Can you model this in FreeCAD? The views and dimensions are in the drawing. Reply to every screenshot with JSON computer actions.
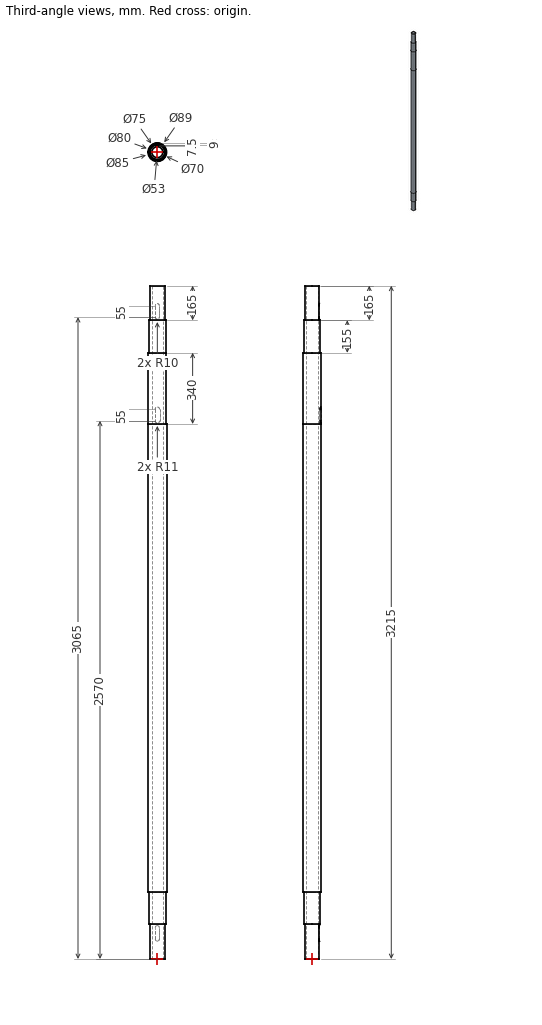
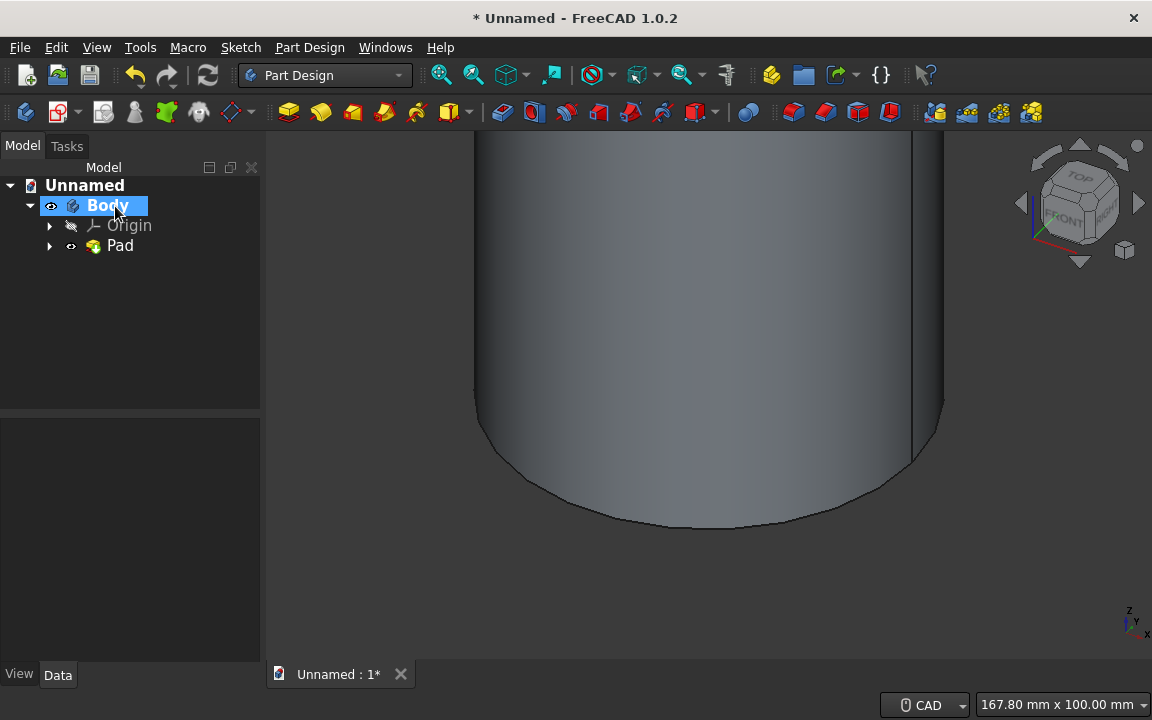
{"action": "left_click", "coordinate": [442, 76]}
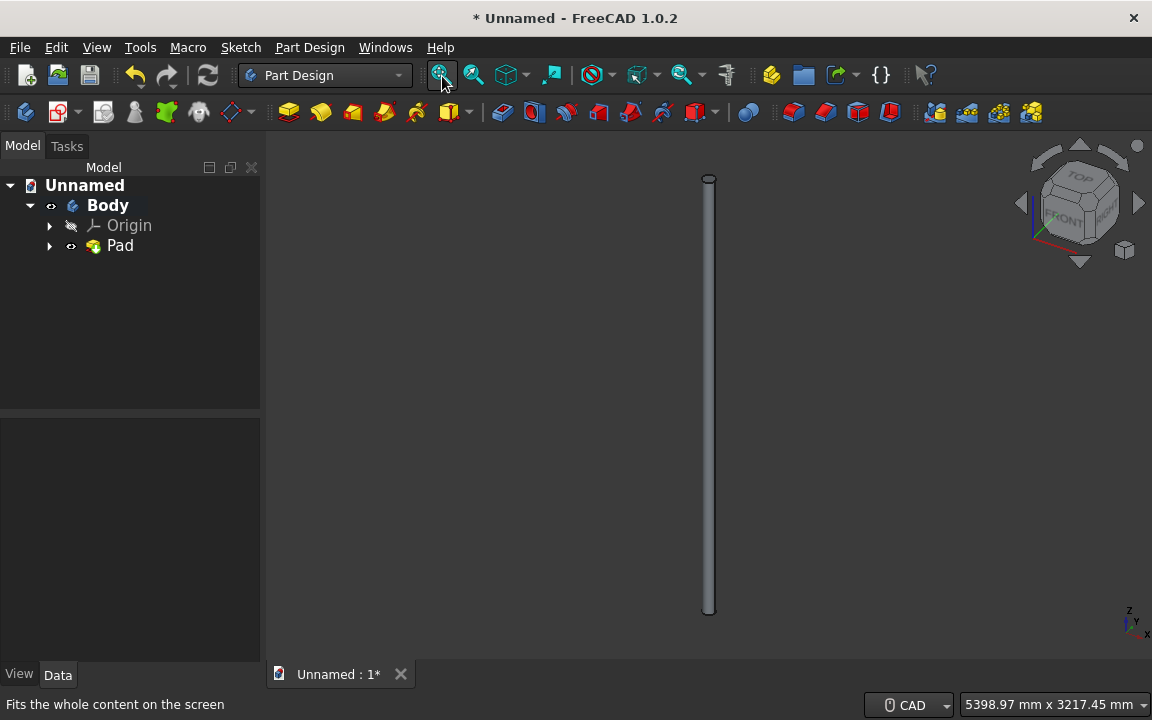
{"action": "left_click", "coordinate": [50, 226]}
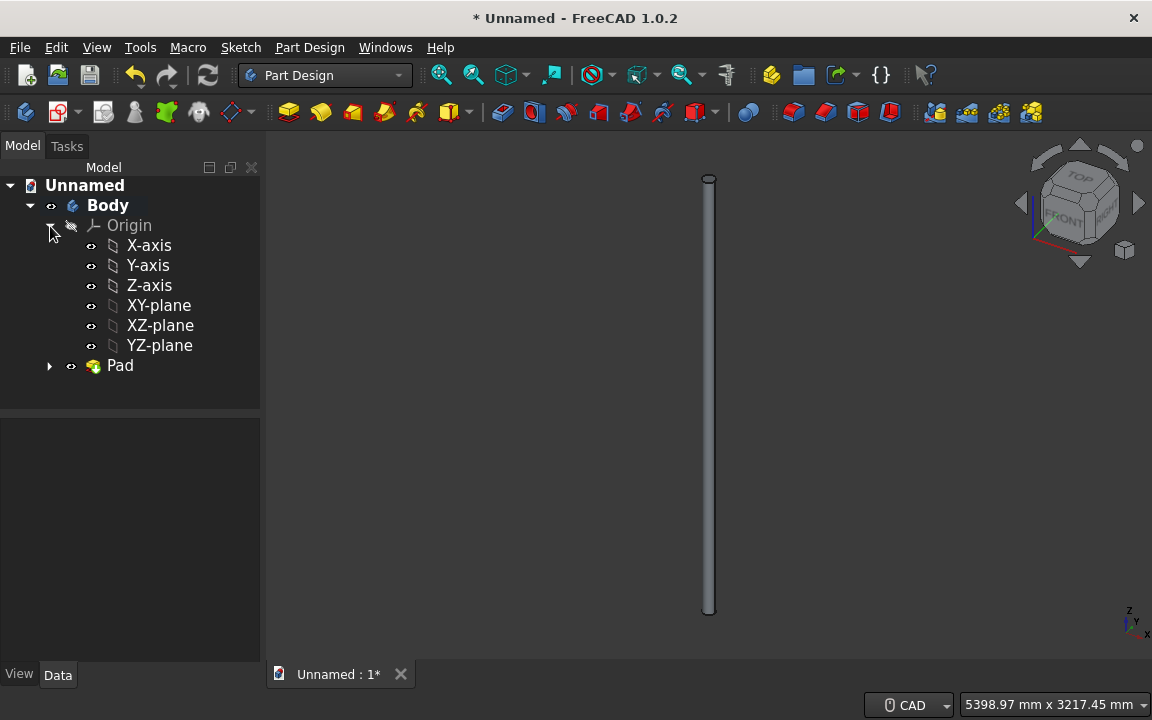
{"action": "left_click", "coordinate": [136, 306]}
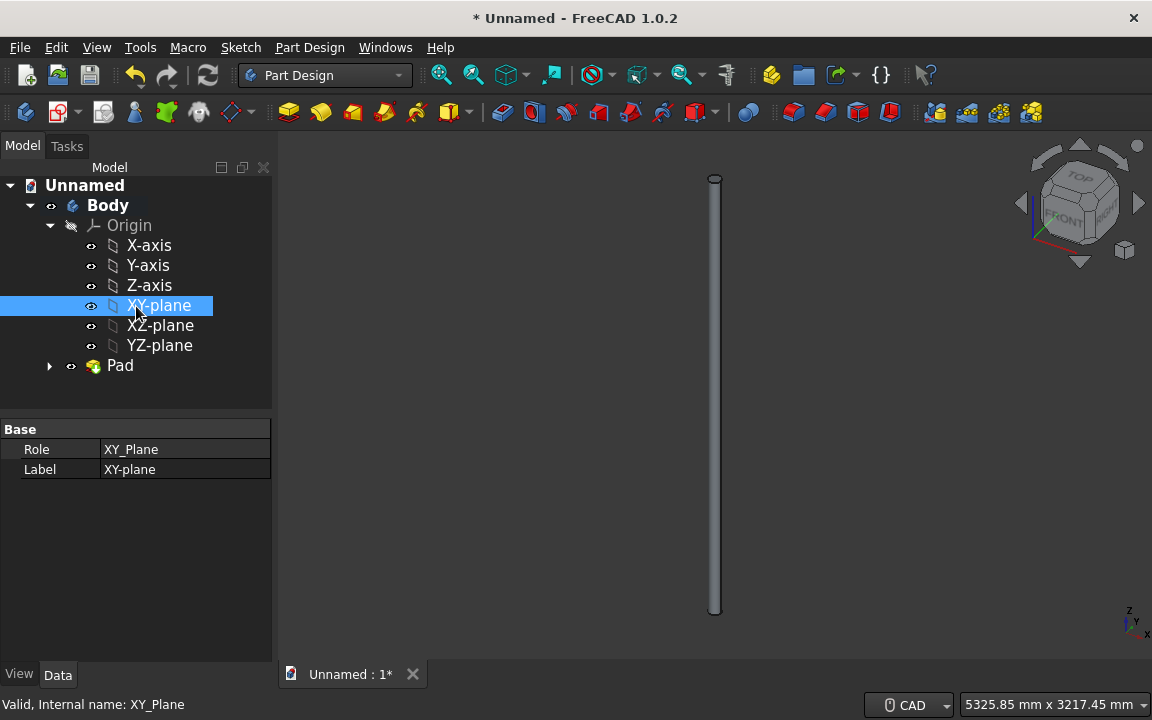
{"action": "left_click", "coordinate": [232, 112]}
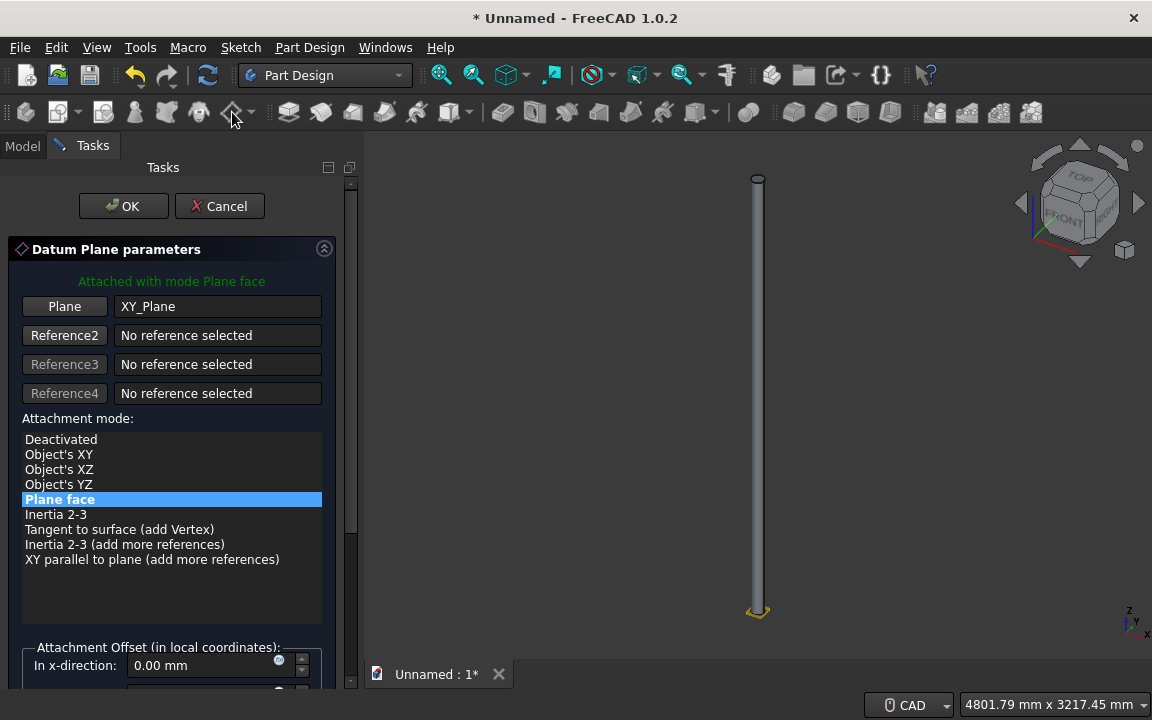
{"action": "scroll", "coordinate": [351, 432], "scroll_direction": "down", "scroll_amount": 2}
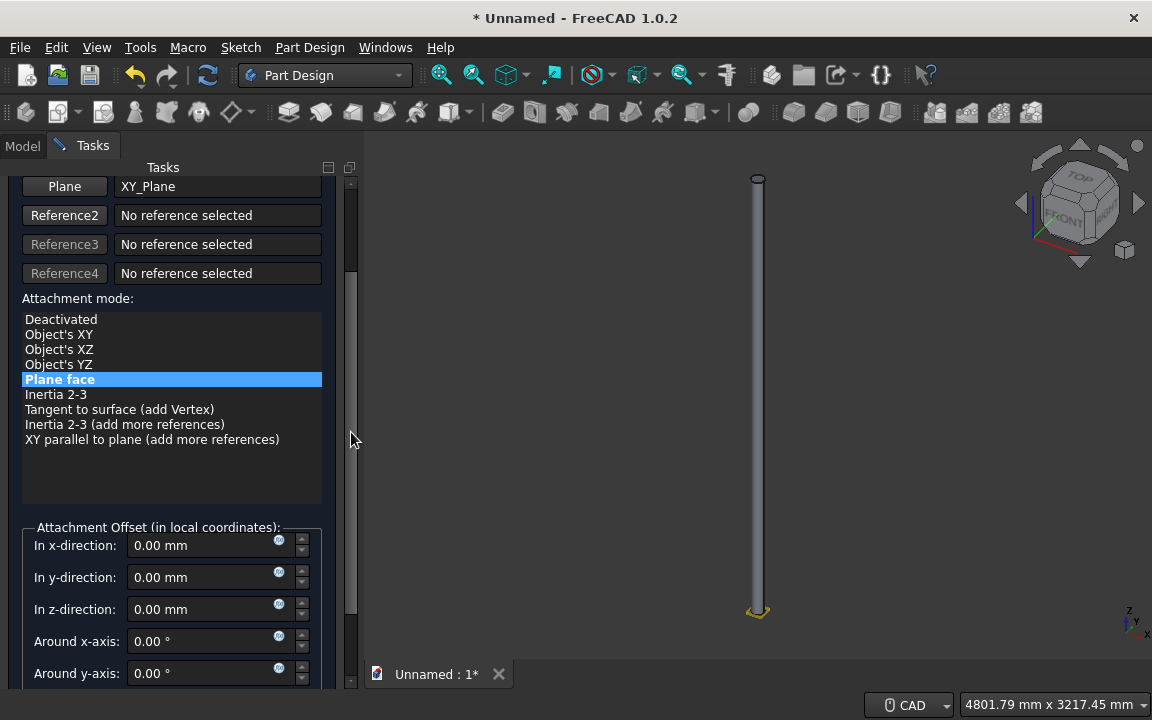
{"action": "triple_click", "coordinate": [210, 609]}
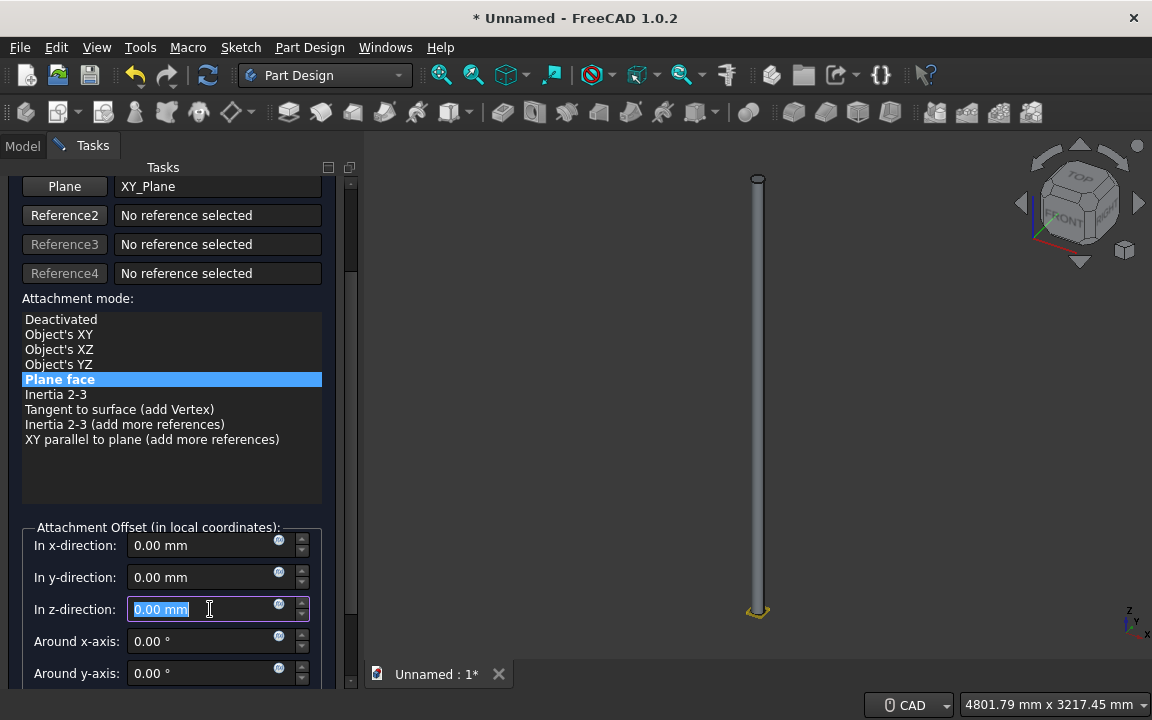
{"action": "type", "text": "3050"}
{"action": "key", "text": "Tab"}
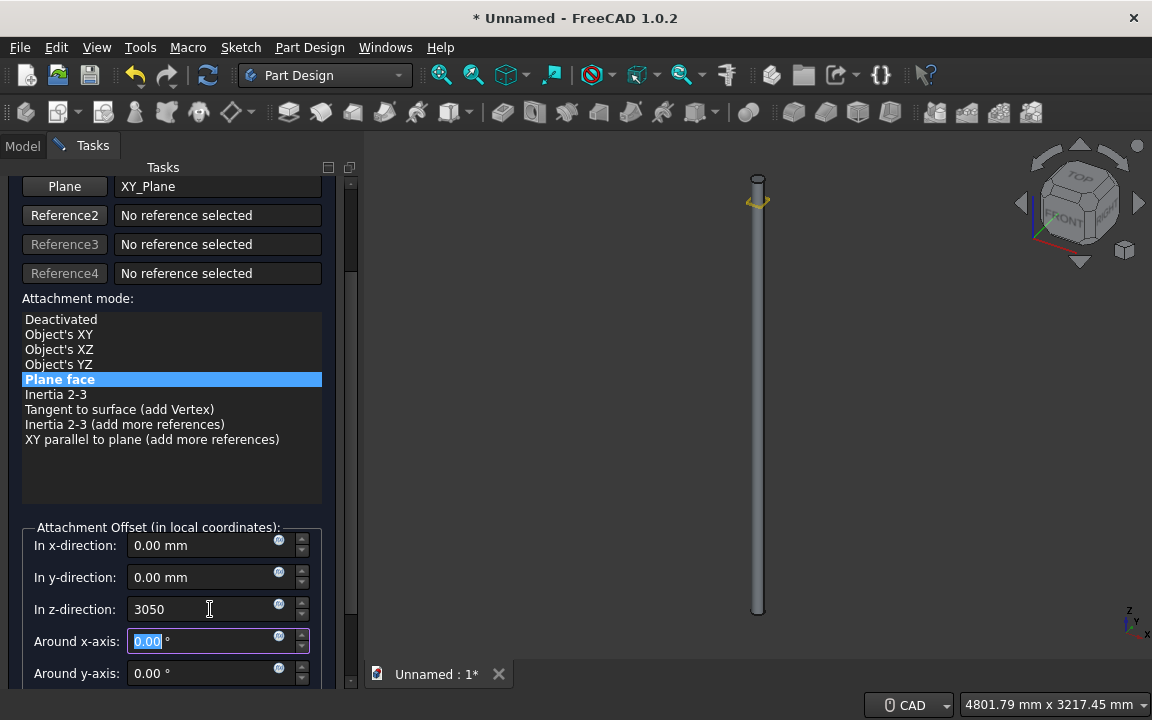
{"action": "scroll", "coordinate": [351, 432], "scroll_direction": "up", "scroll_amount": 3}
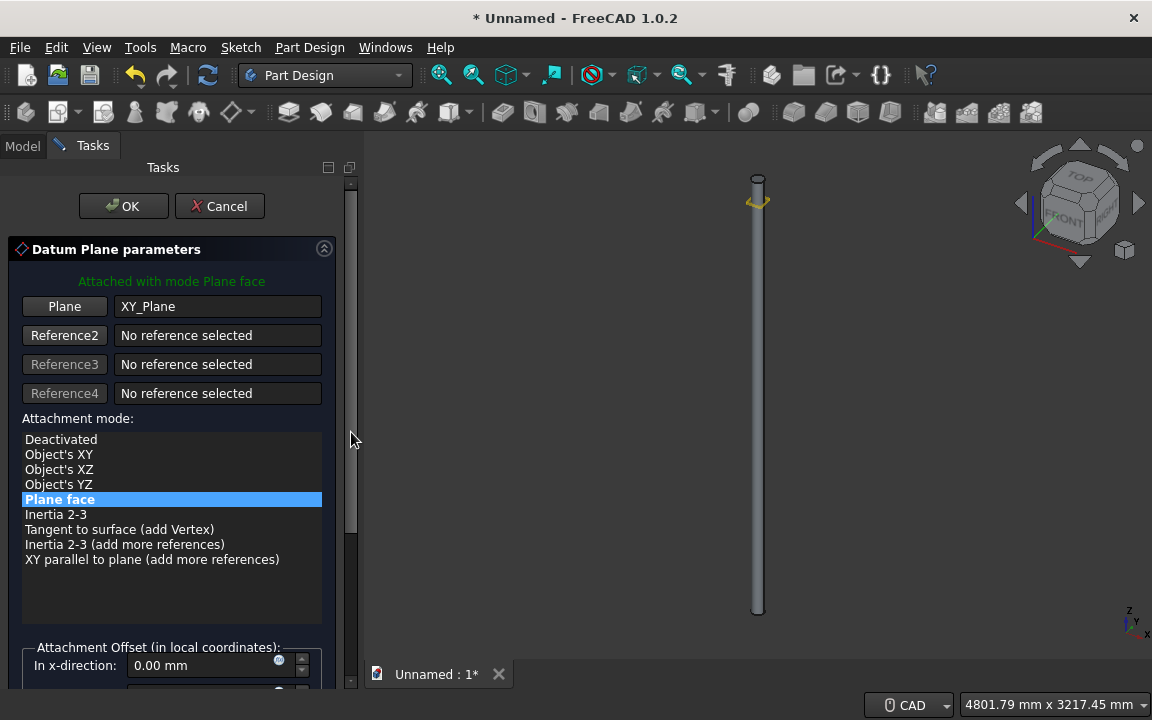
{"action": "left_click", "coordinate": [124, 206]}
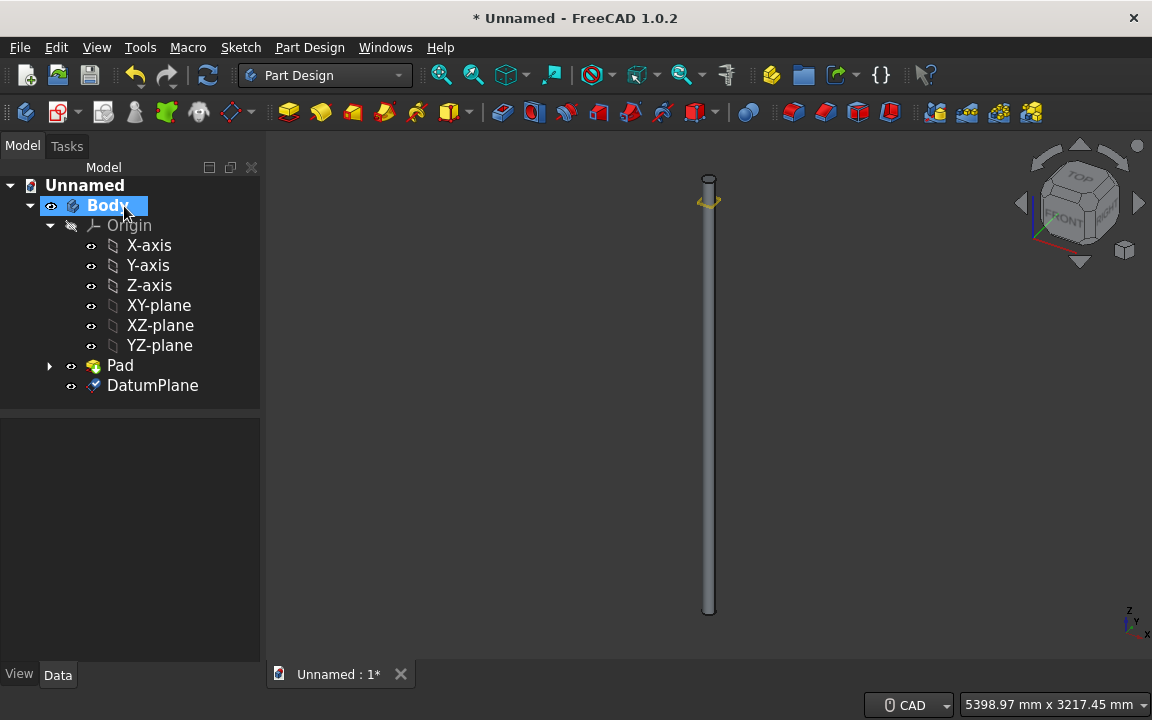
{"action": "left_click", "coordinate": [116, 386]}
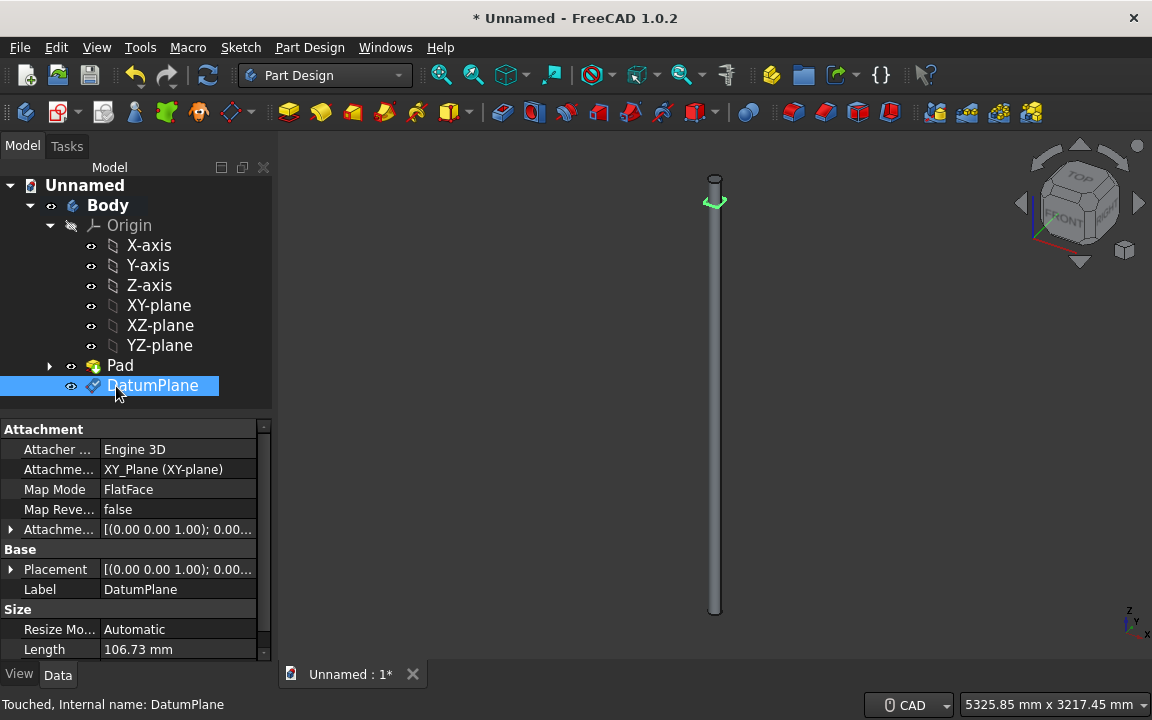
{"action": "left_click", "coordinate": [58, 112]}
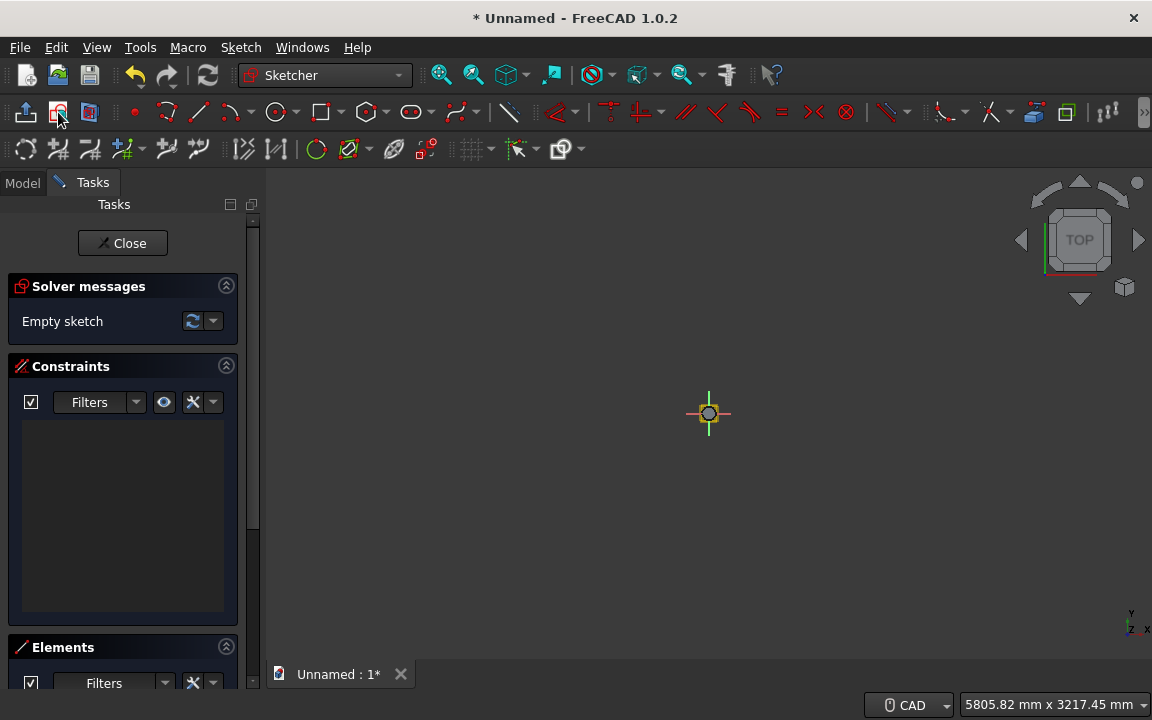
{"action": "left_click", "coordinate": [90, 112]}